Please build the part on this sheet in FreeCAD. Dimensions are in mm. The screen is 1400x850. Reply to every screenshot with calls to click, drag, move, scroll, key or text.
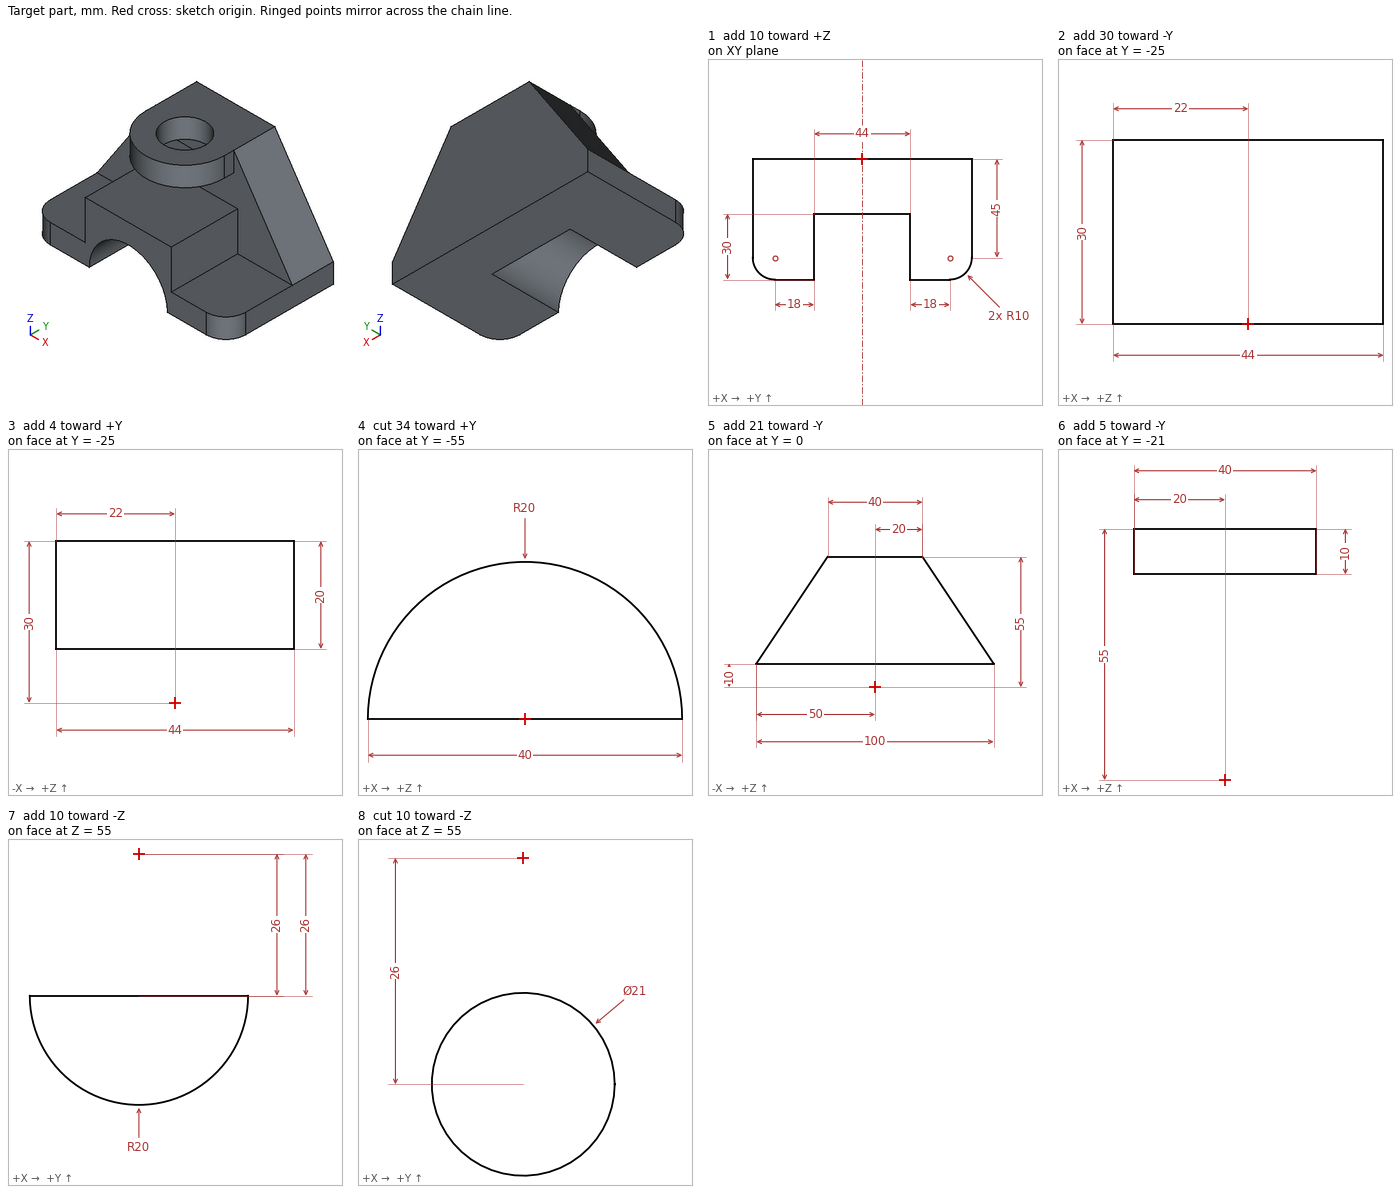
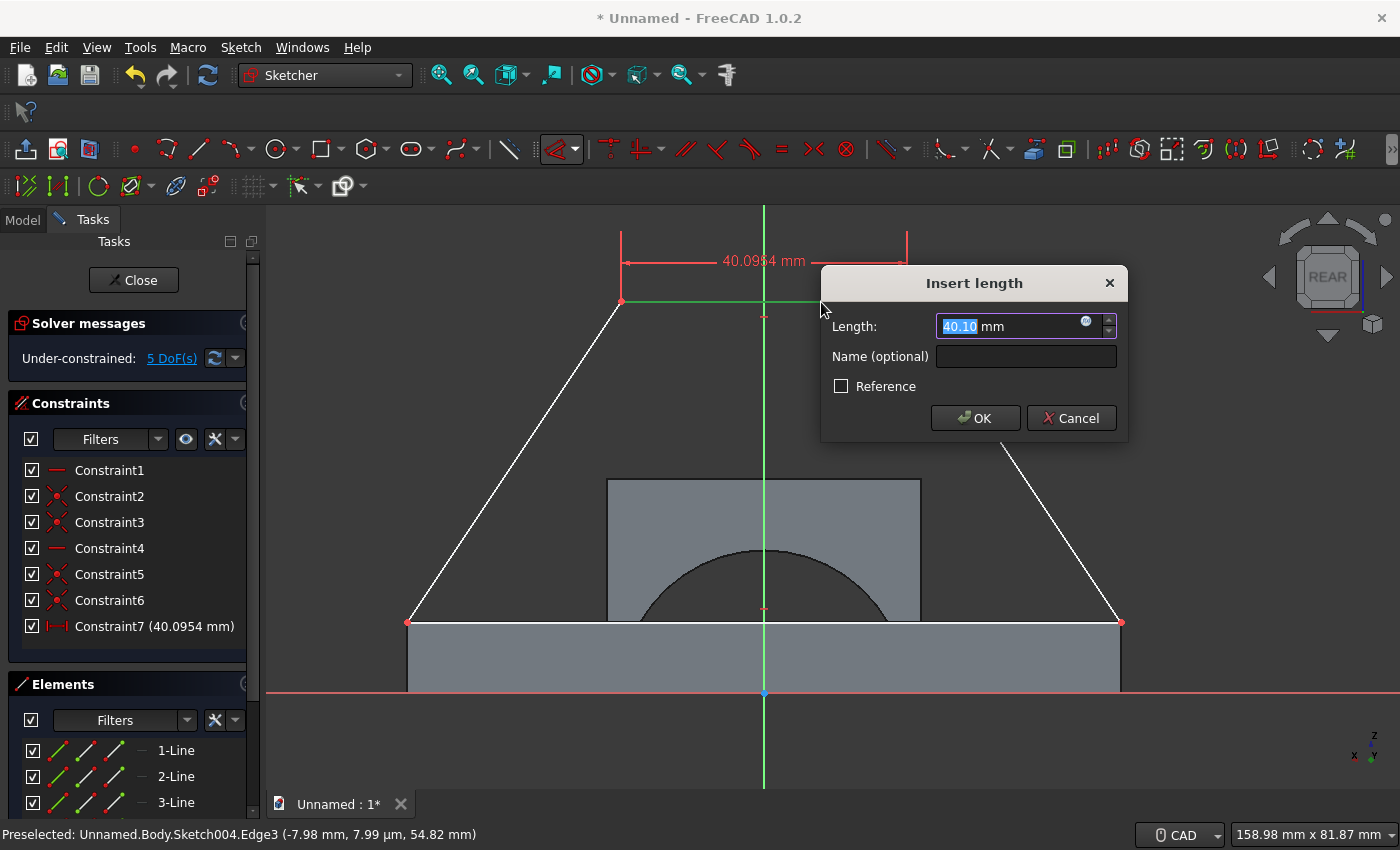
text(40)
key(Return)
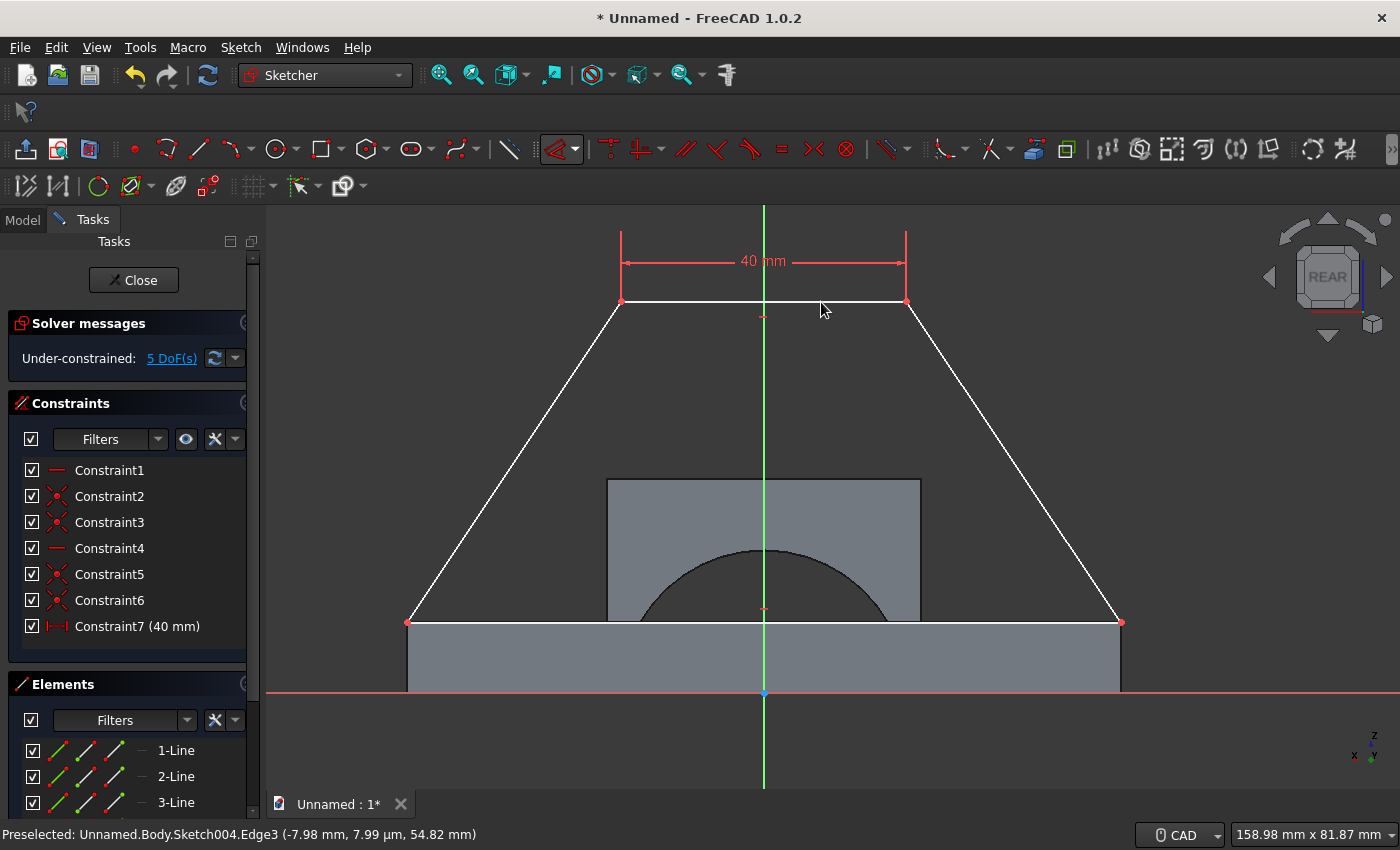
click(621, 623)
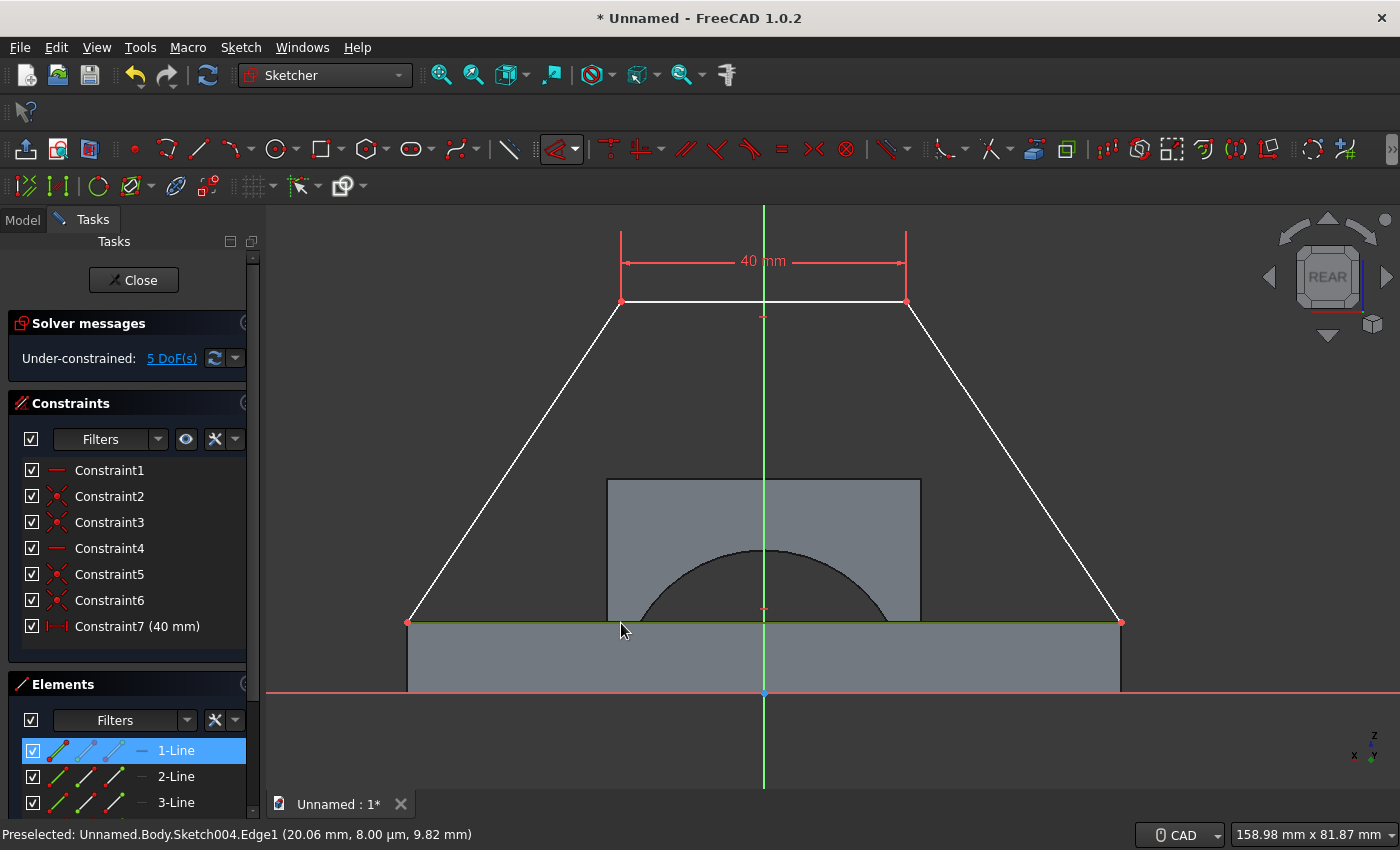
key(l)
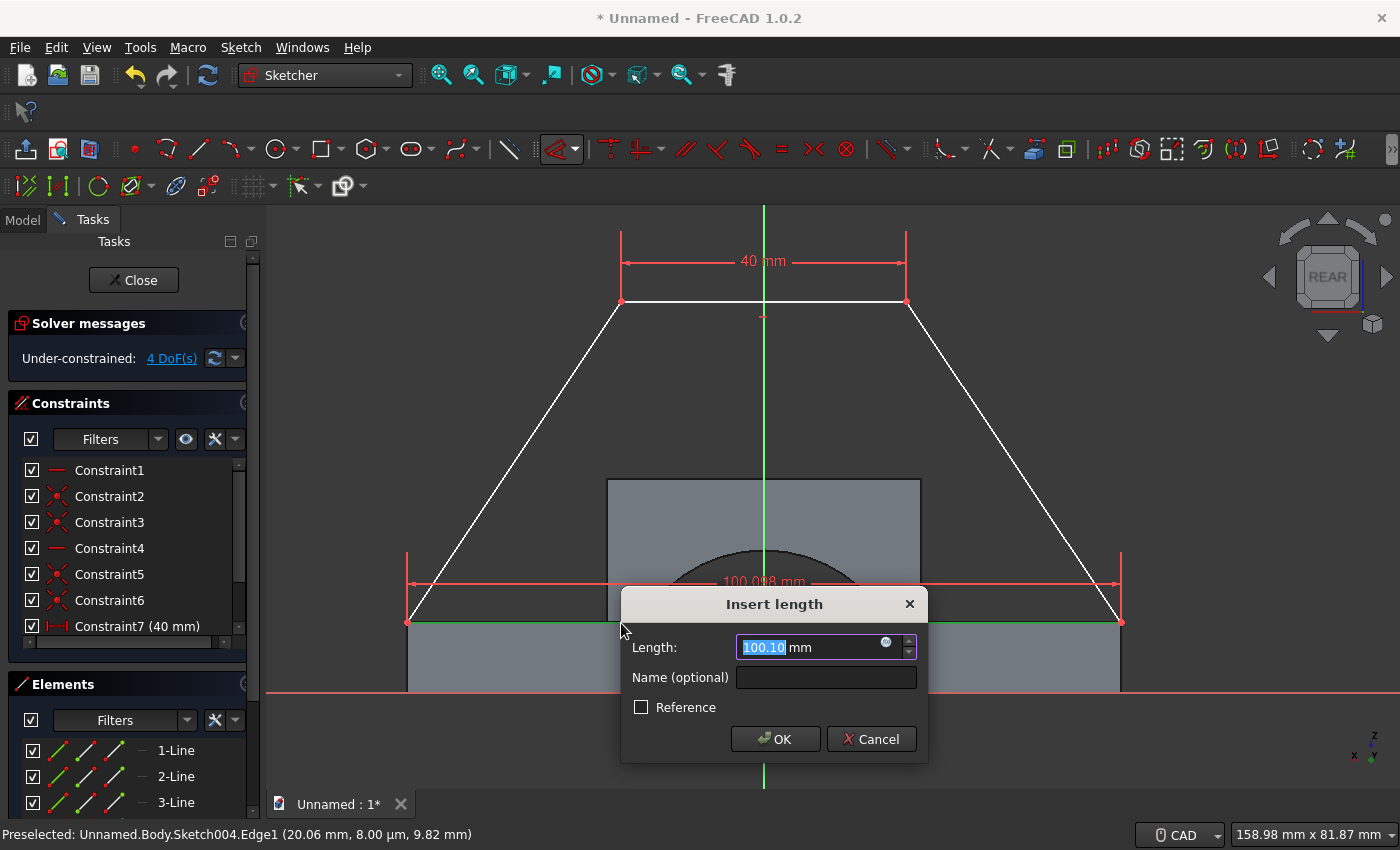
text(100)
key(Return)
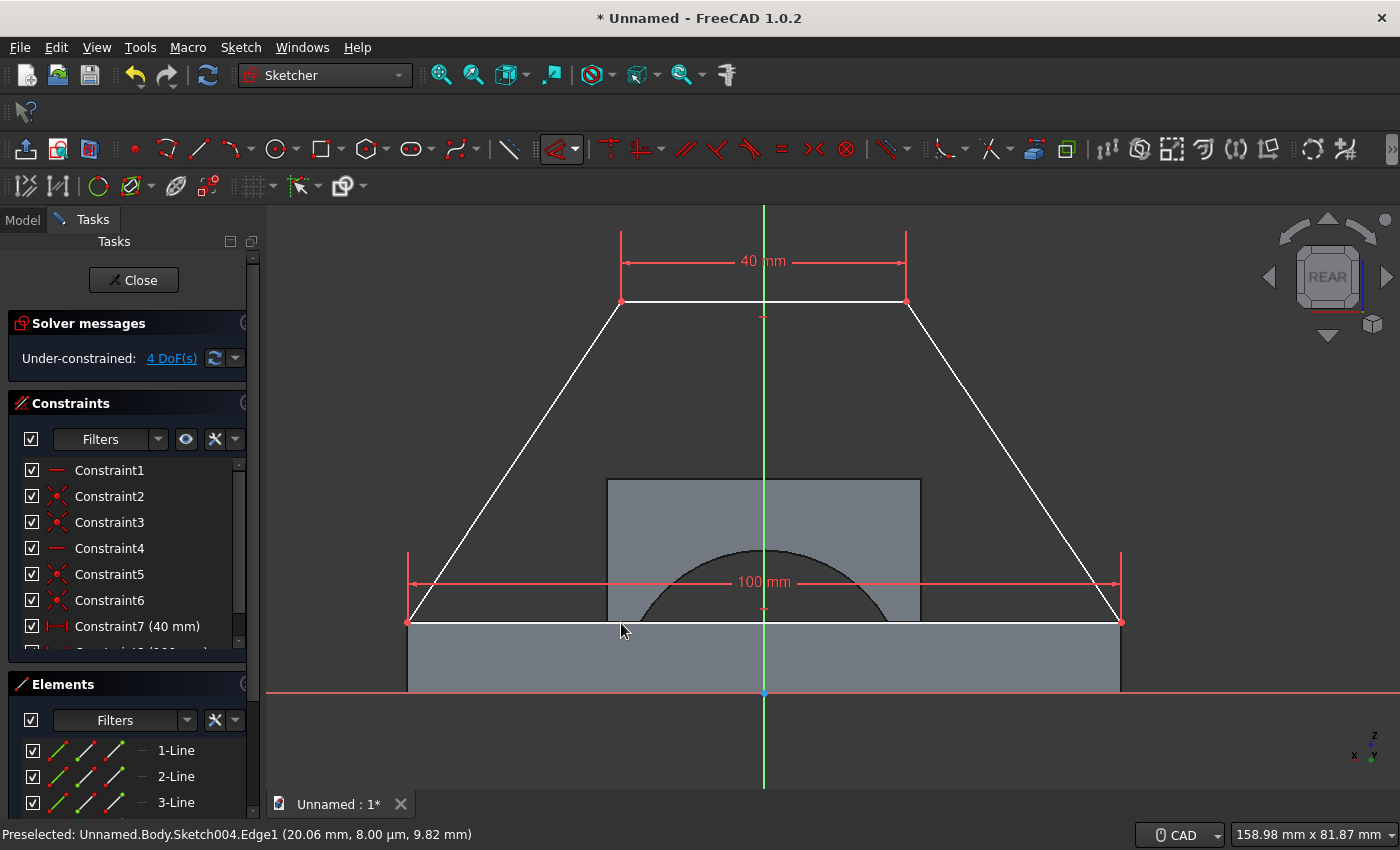
click(408, 623)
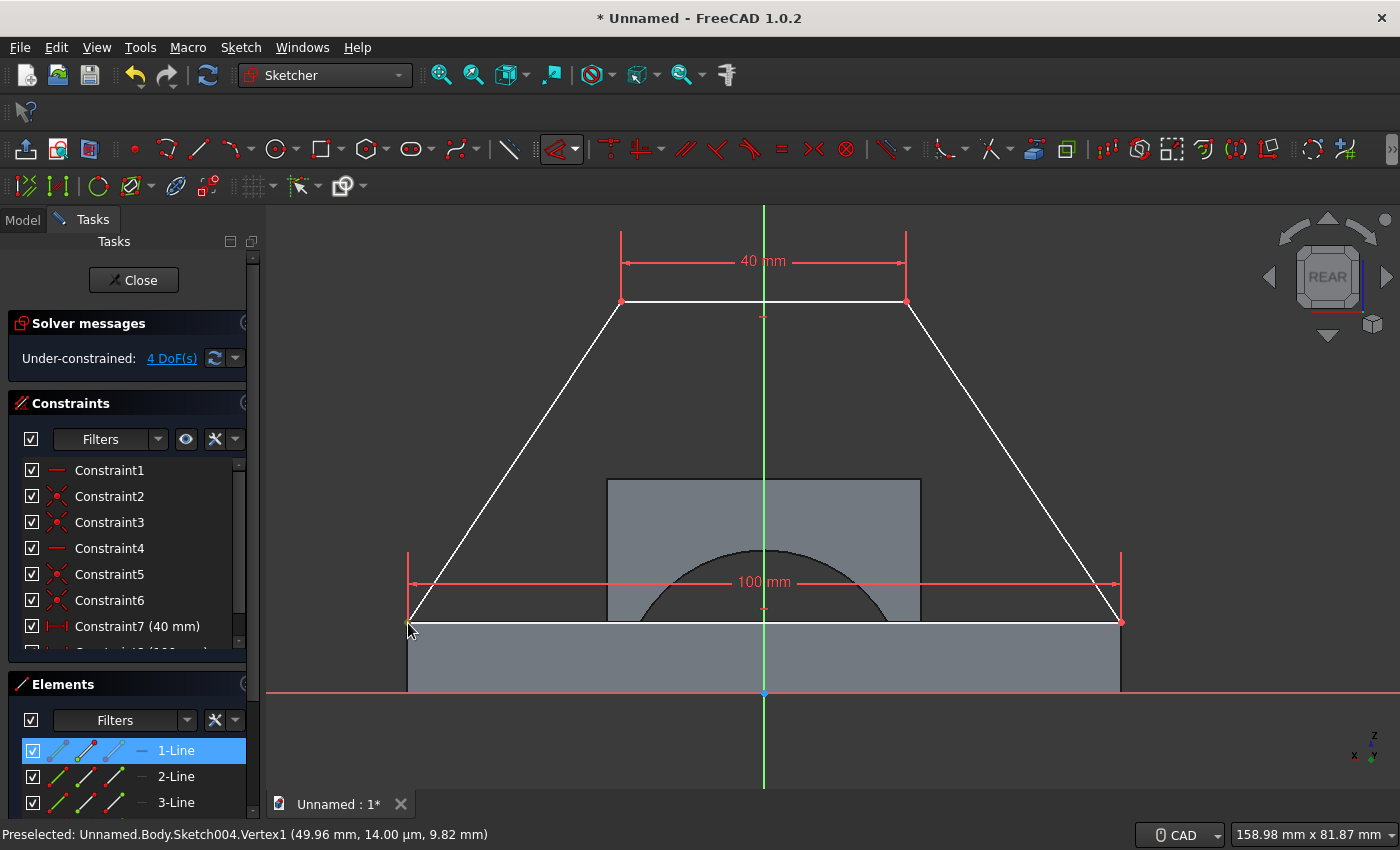
click(578, 150)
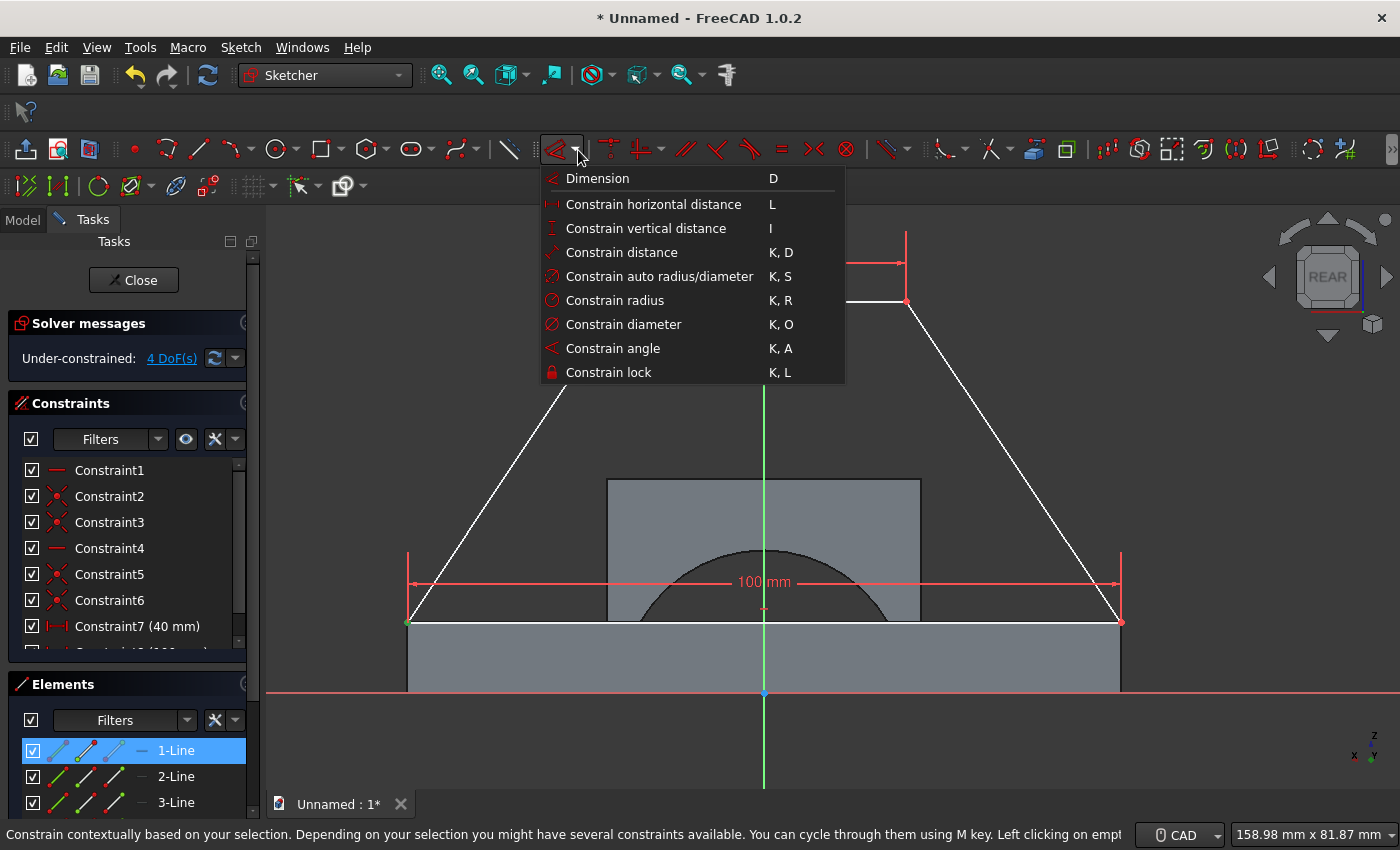
click(693, 204)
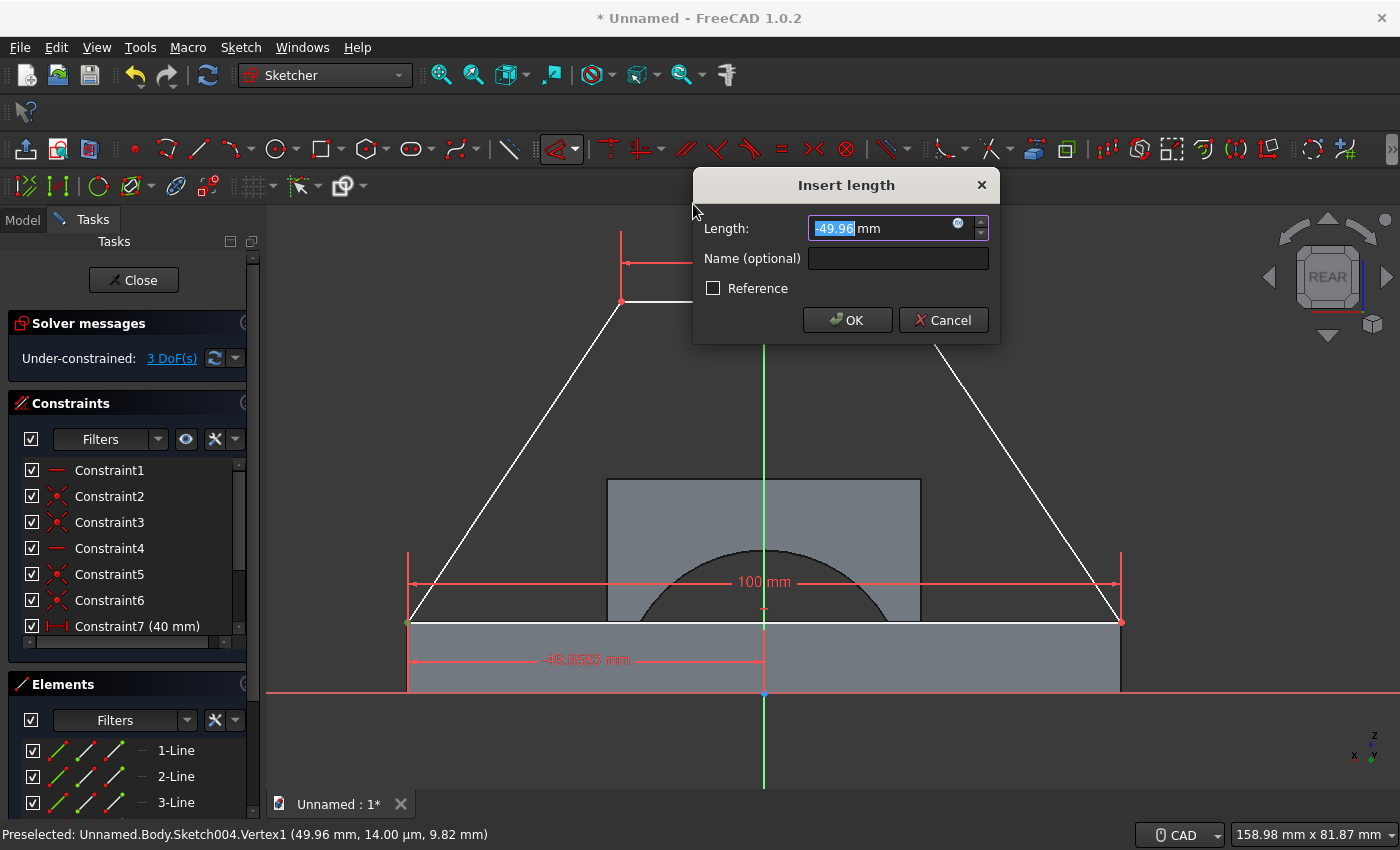
text(-50)
key(Return)